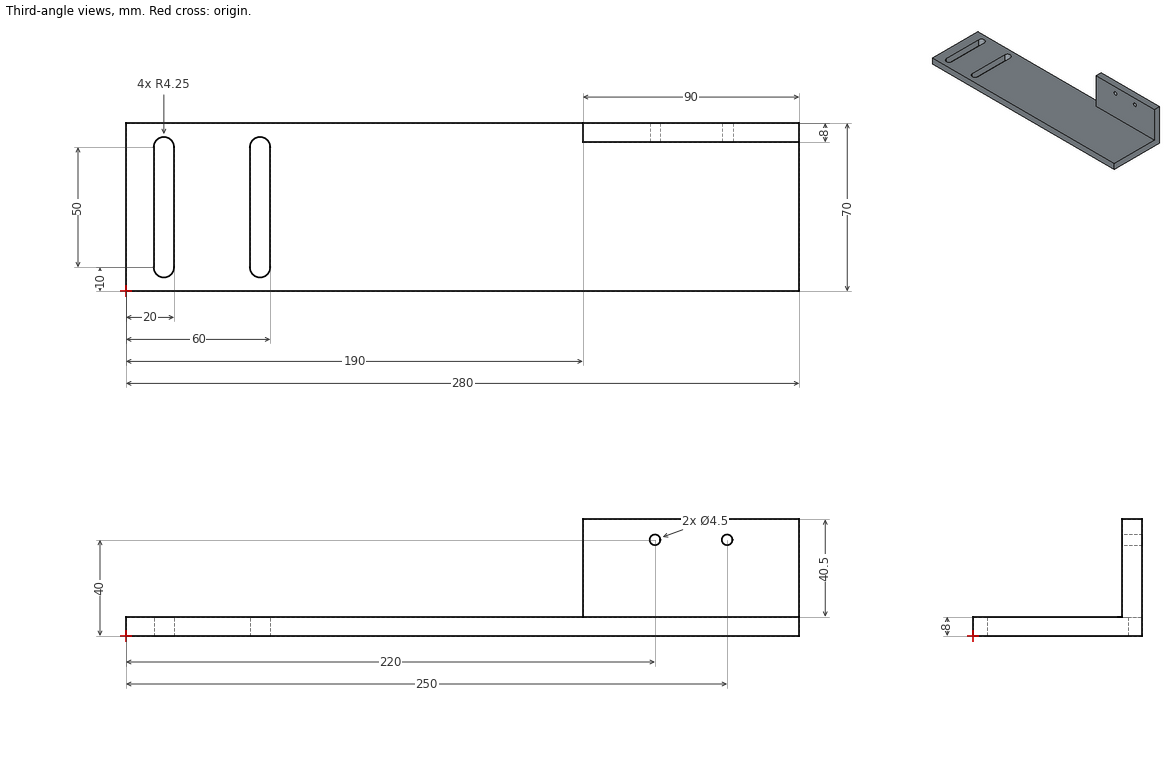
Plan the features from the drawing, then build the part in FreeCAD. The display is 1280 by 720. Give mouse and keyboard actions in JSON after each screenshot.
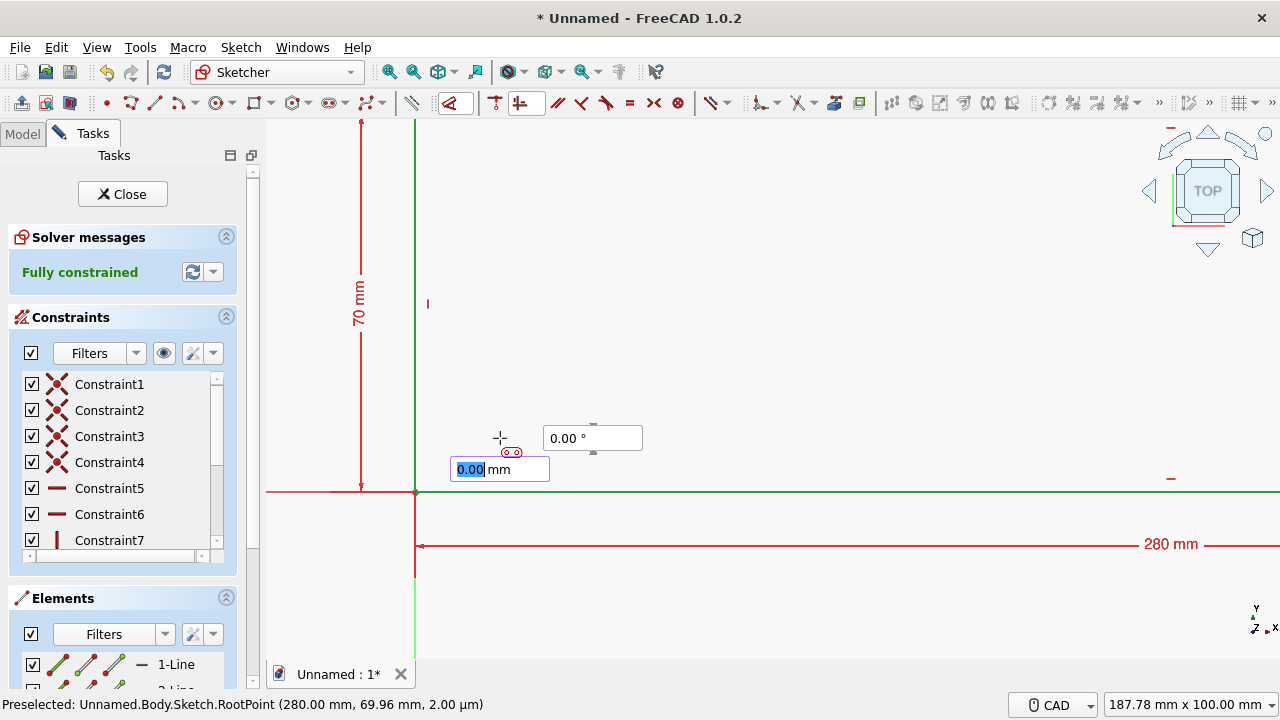
{"action": "left_click", "coordinate": [500, 168]}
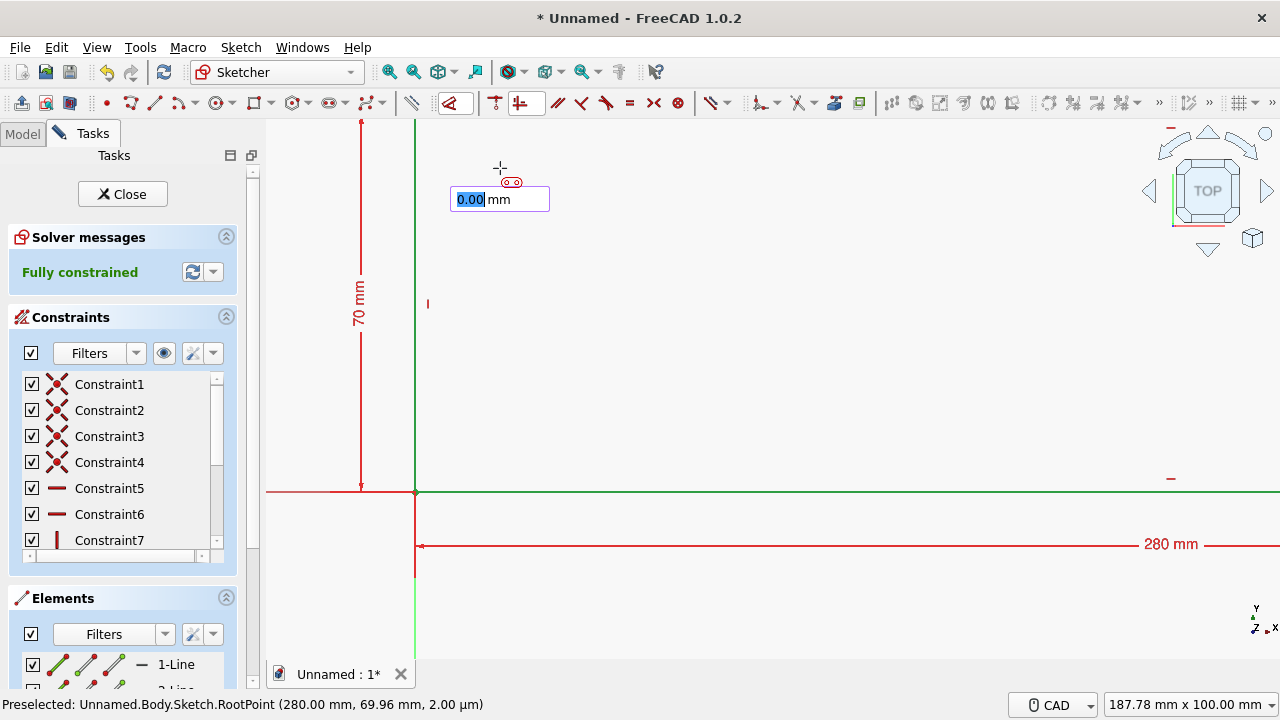
{"action": "left_click", "coordinate": [477, 303]}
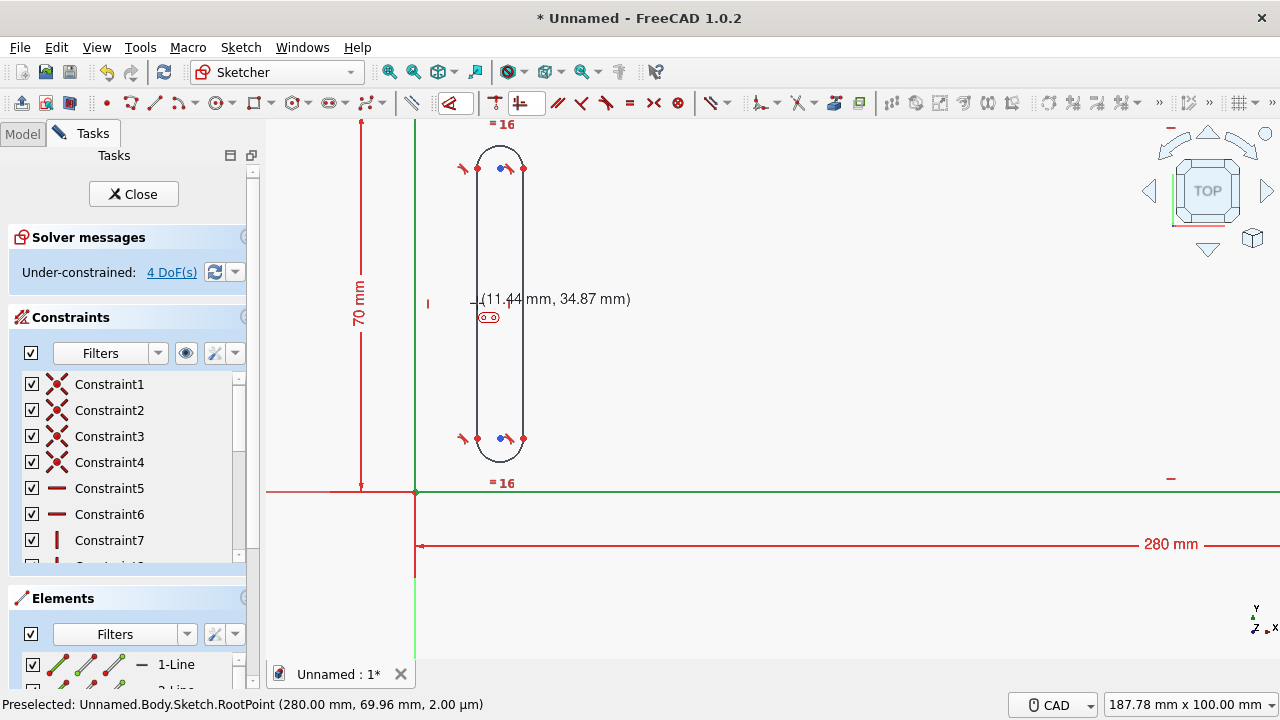
{"action": "left_click", "coordinate": [716, 438]}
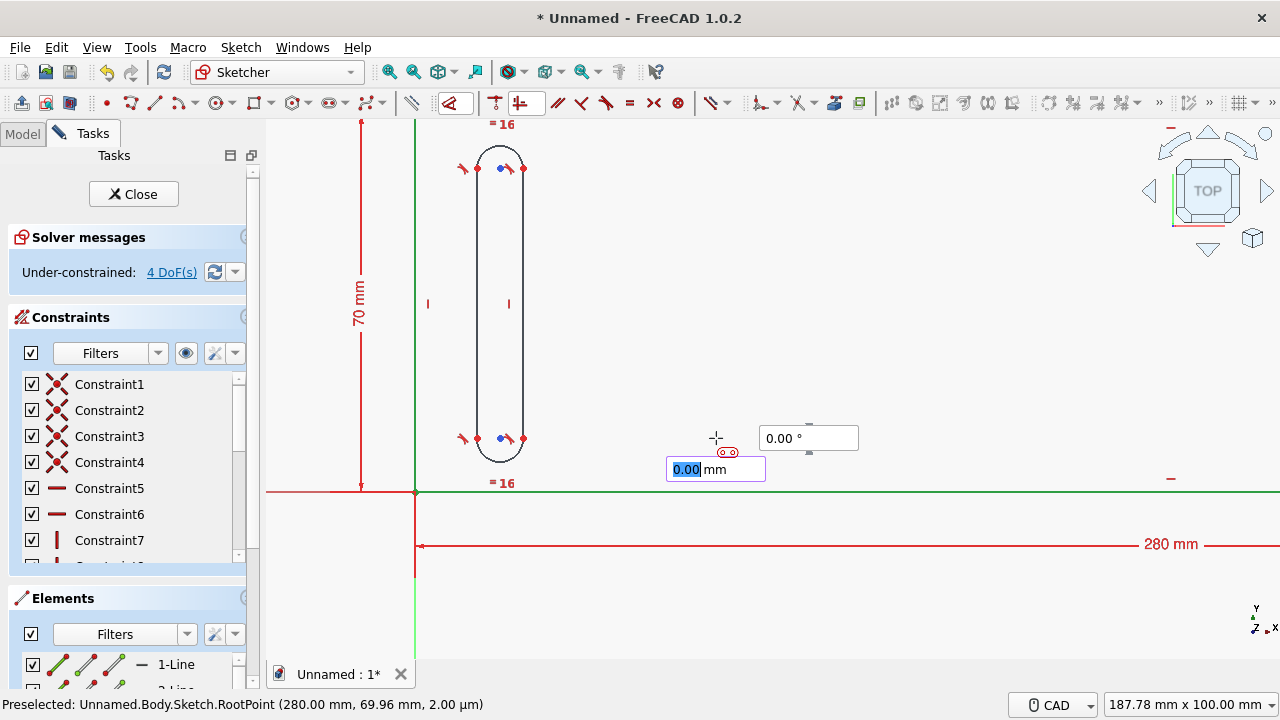
{"action": "left_click", "coordinate": [716, 168]}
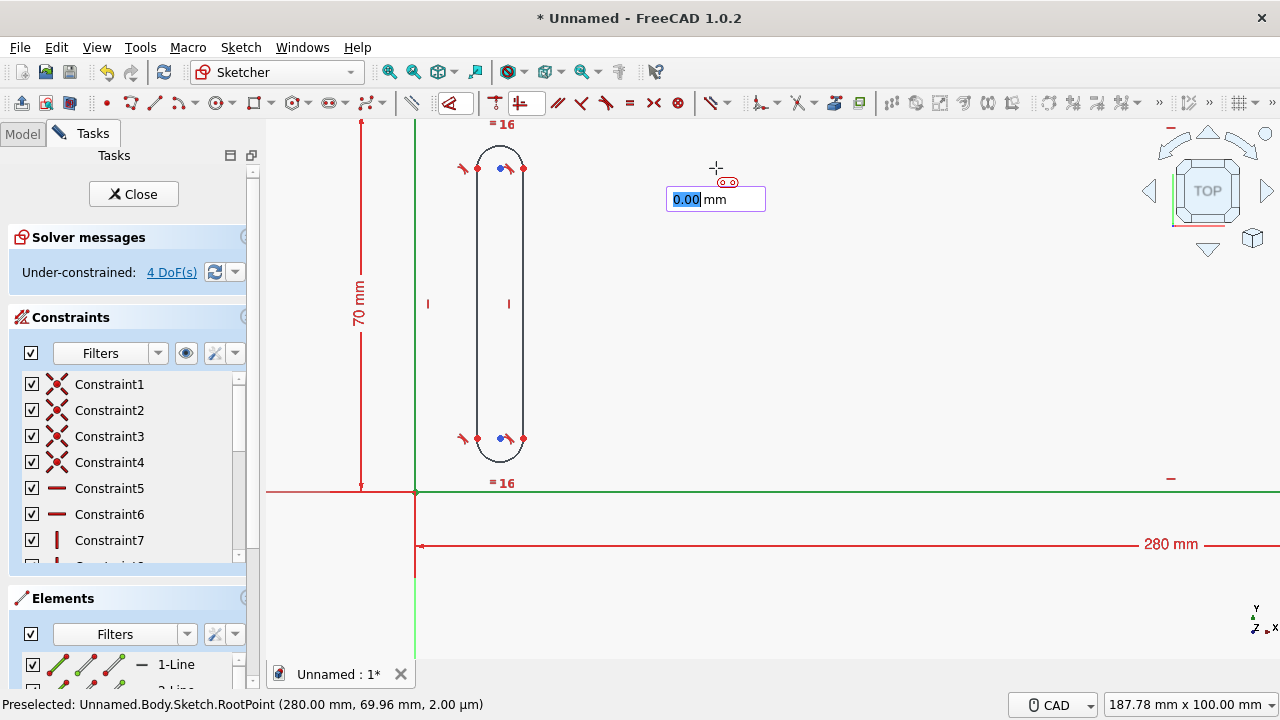
{"action": "left_click", "coordinate": [693, 303]}
{"action": "key", "text": "Escape"}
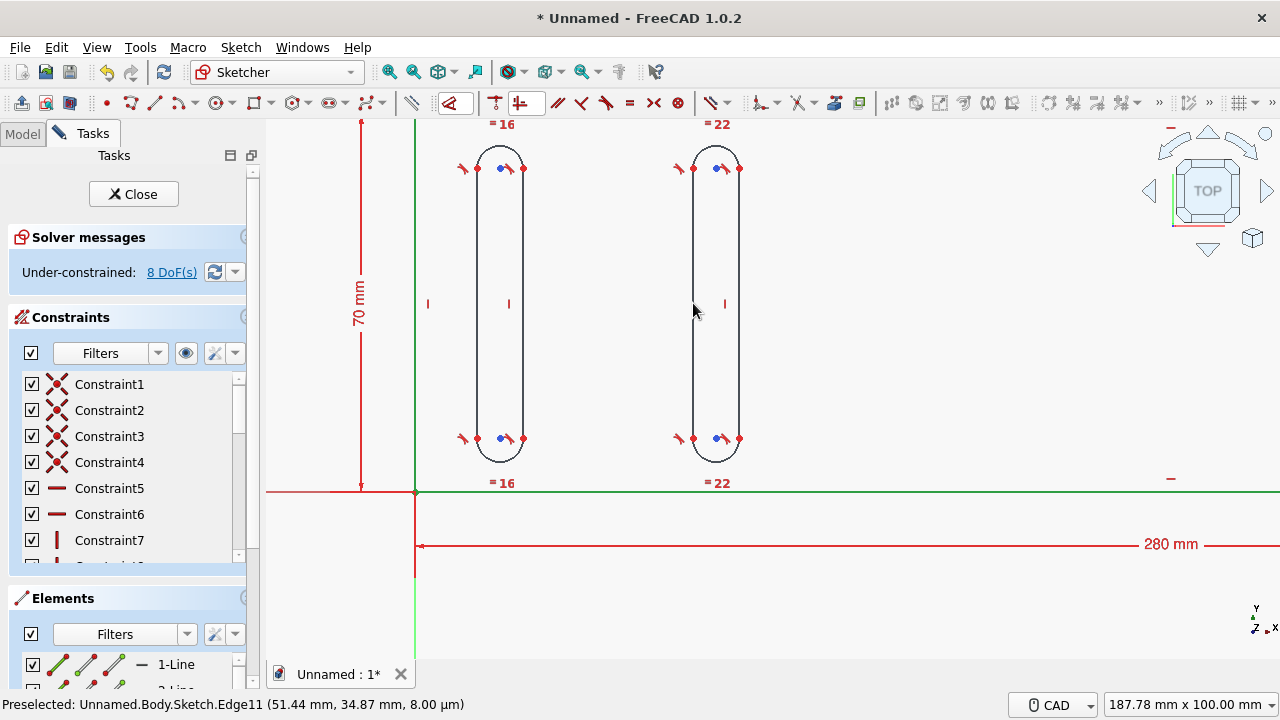
{"action": "left_click", "coordinate": [486, 458]}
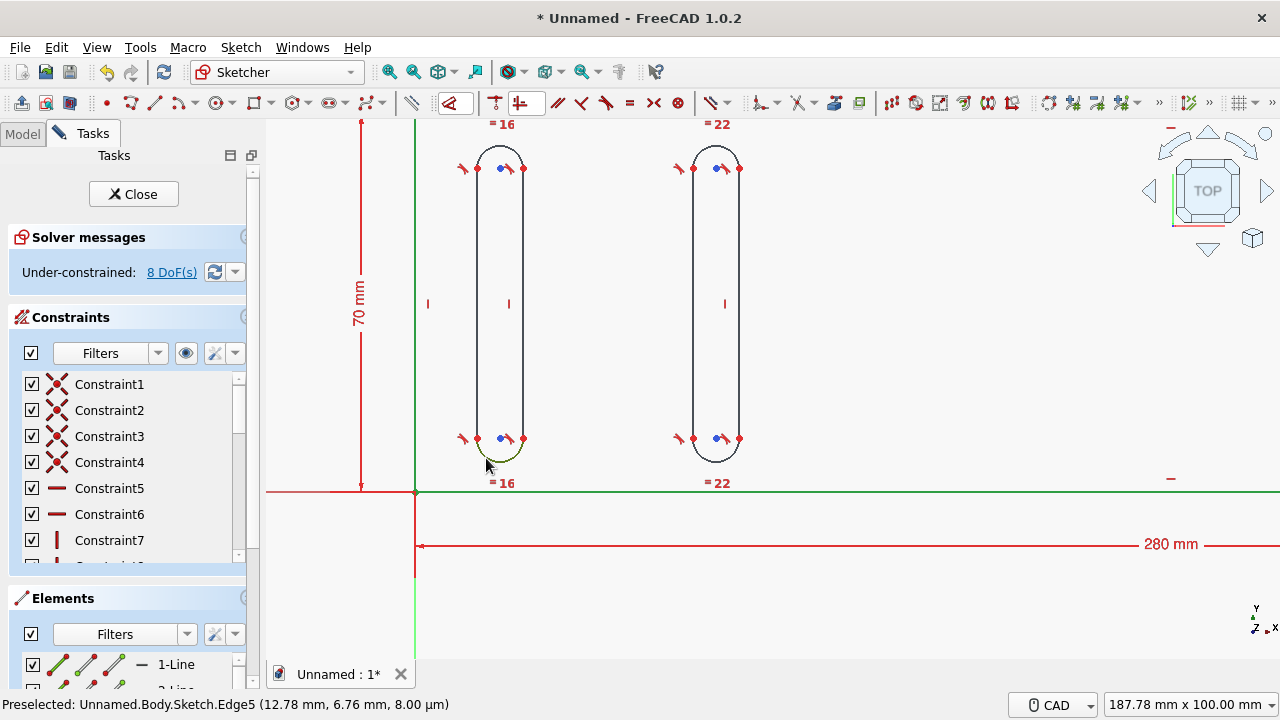
{"action": "left_click", "coordinate": [702, 458]}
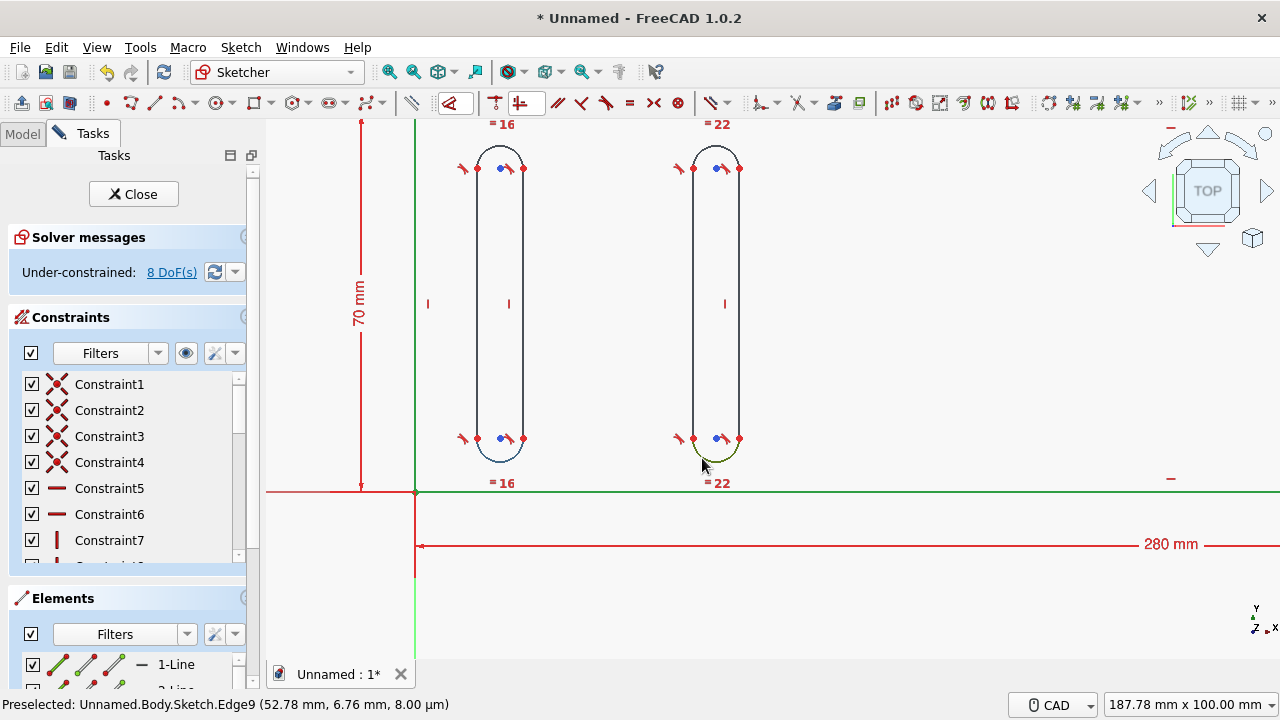
{"action": "key", "text": "e"}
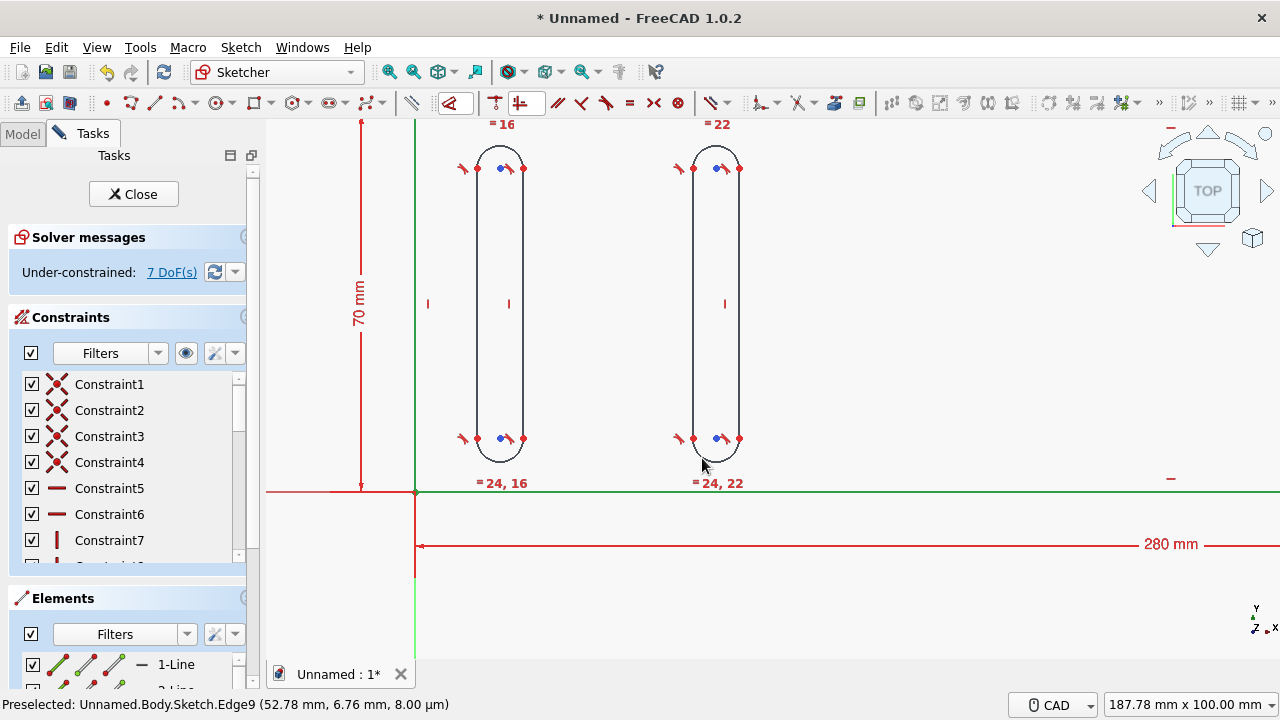
{"action": "scroll", "coordinate": [486, 458], "scroll_direction": "up", "scroll_amount": 3}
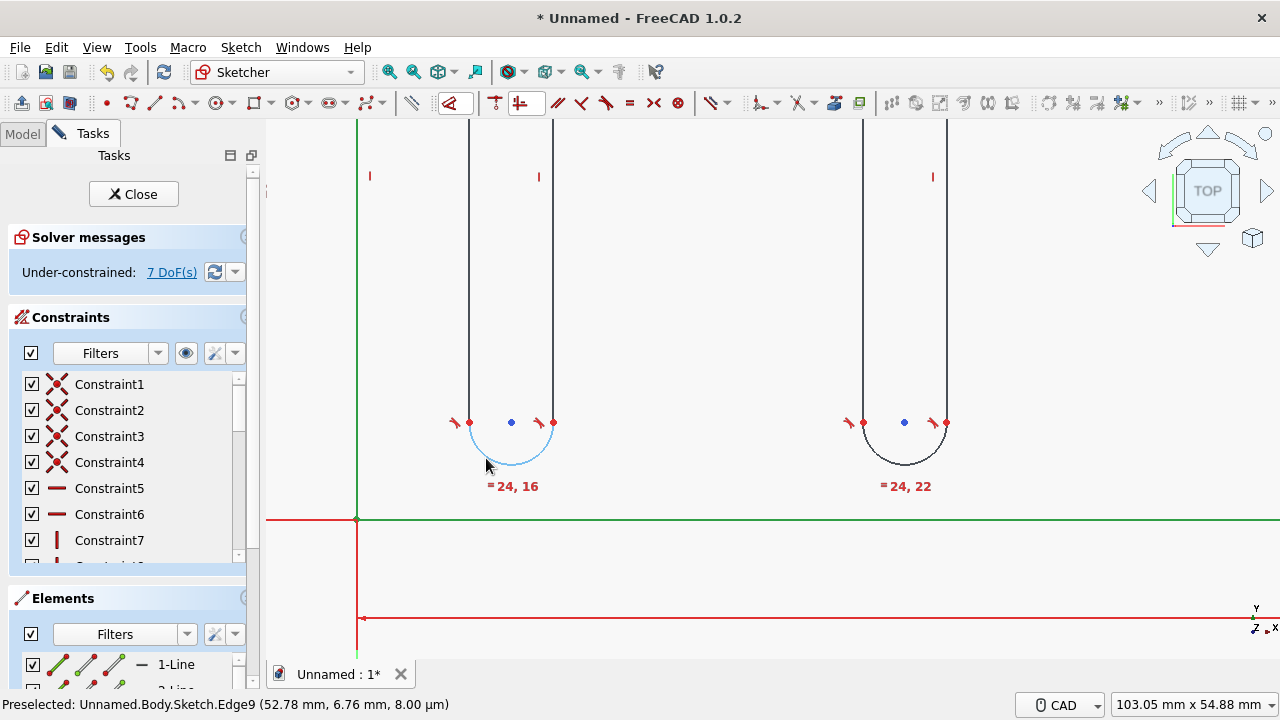
{"action": "left_click", "coordinate": [487, 457]}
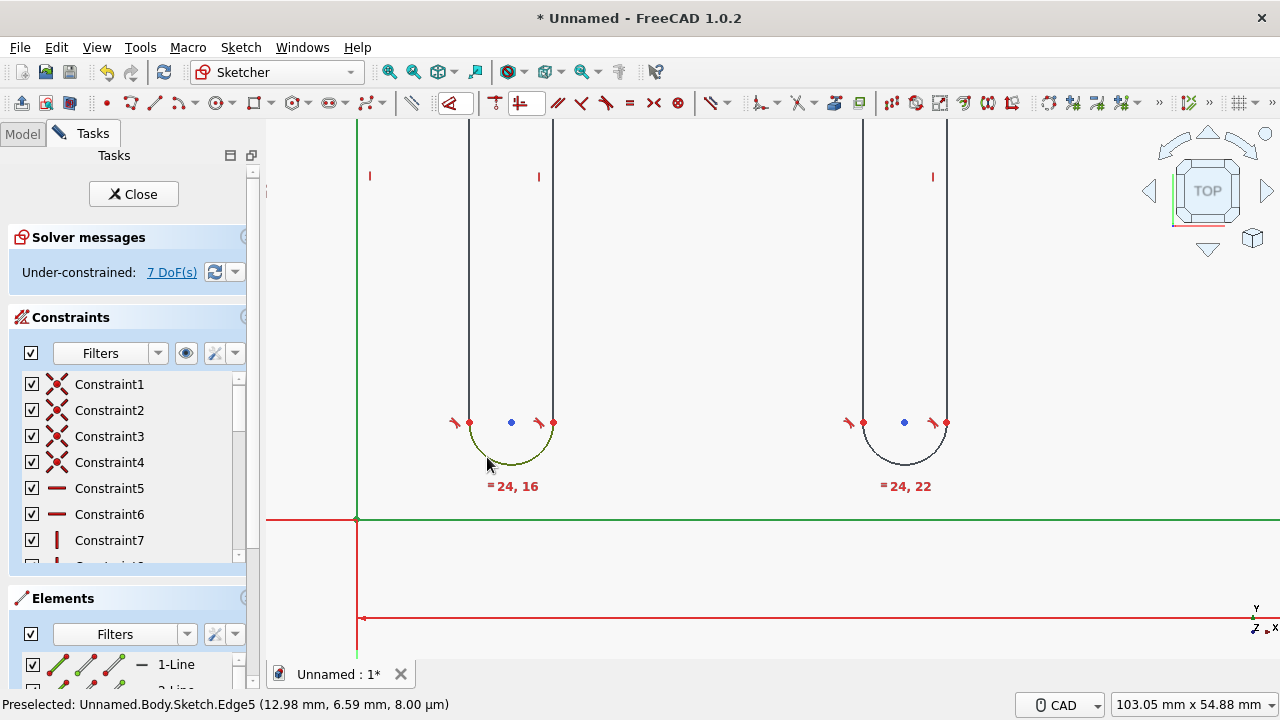
{"action": "left_click", "coordinate": [468, 104]}